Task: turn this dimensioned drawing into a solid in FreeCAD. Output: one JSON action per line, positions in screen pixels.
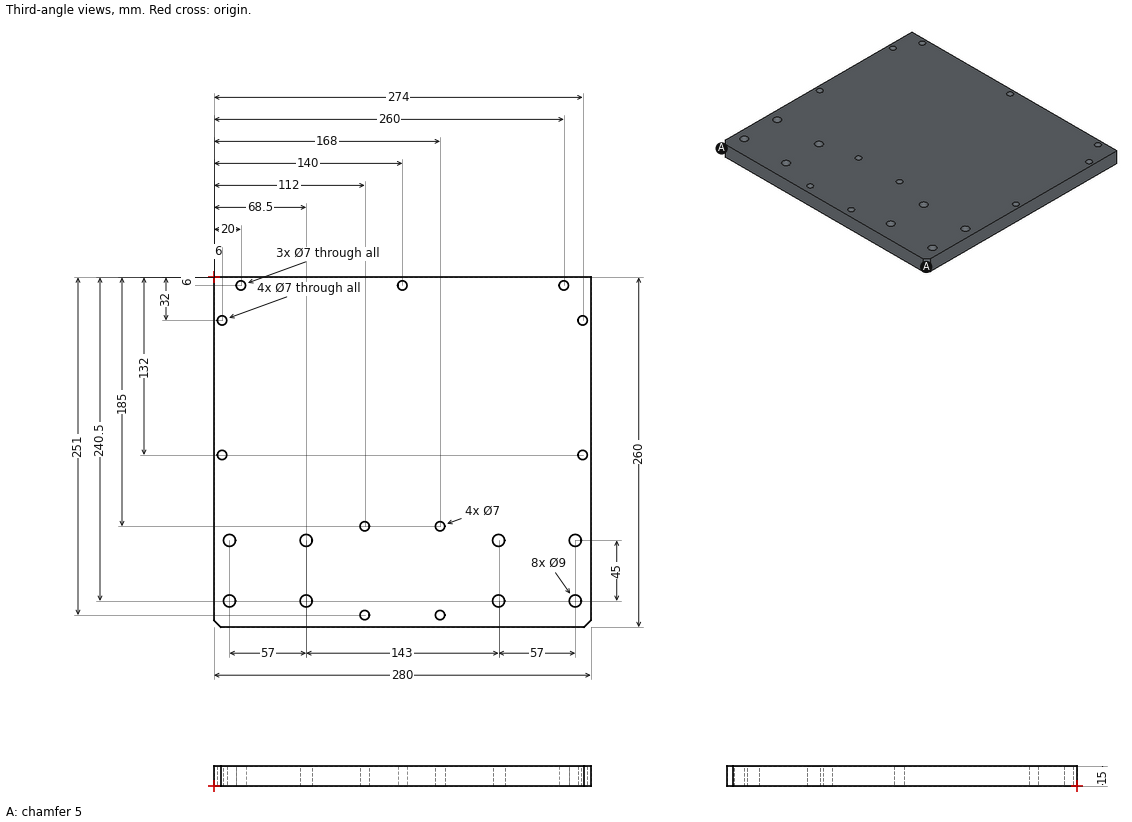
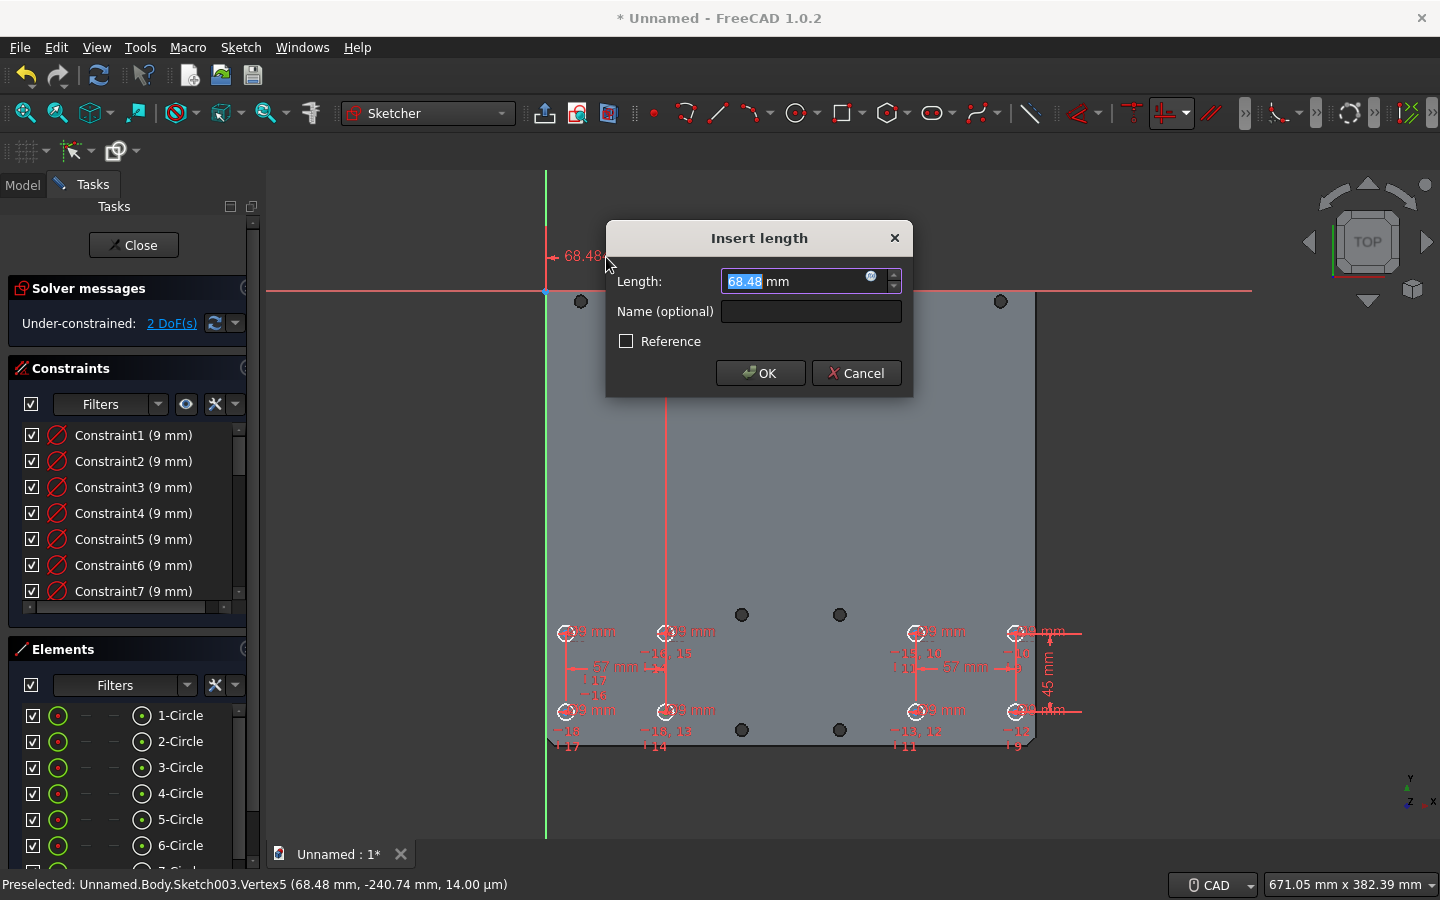
{"action": "type", "text": "68.5"}
{"action": "key", "text": "Return"}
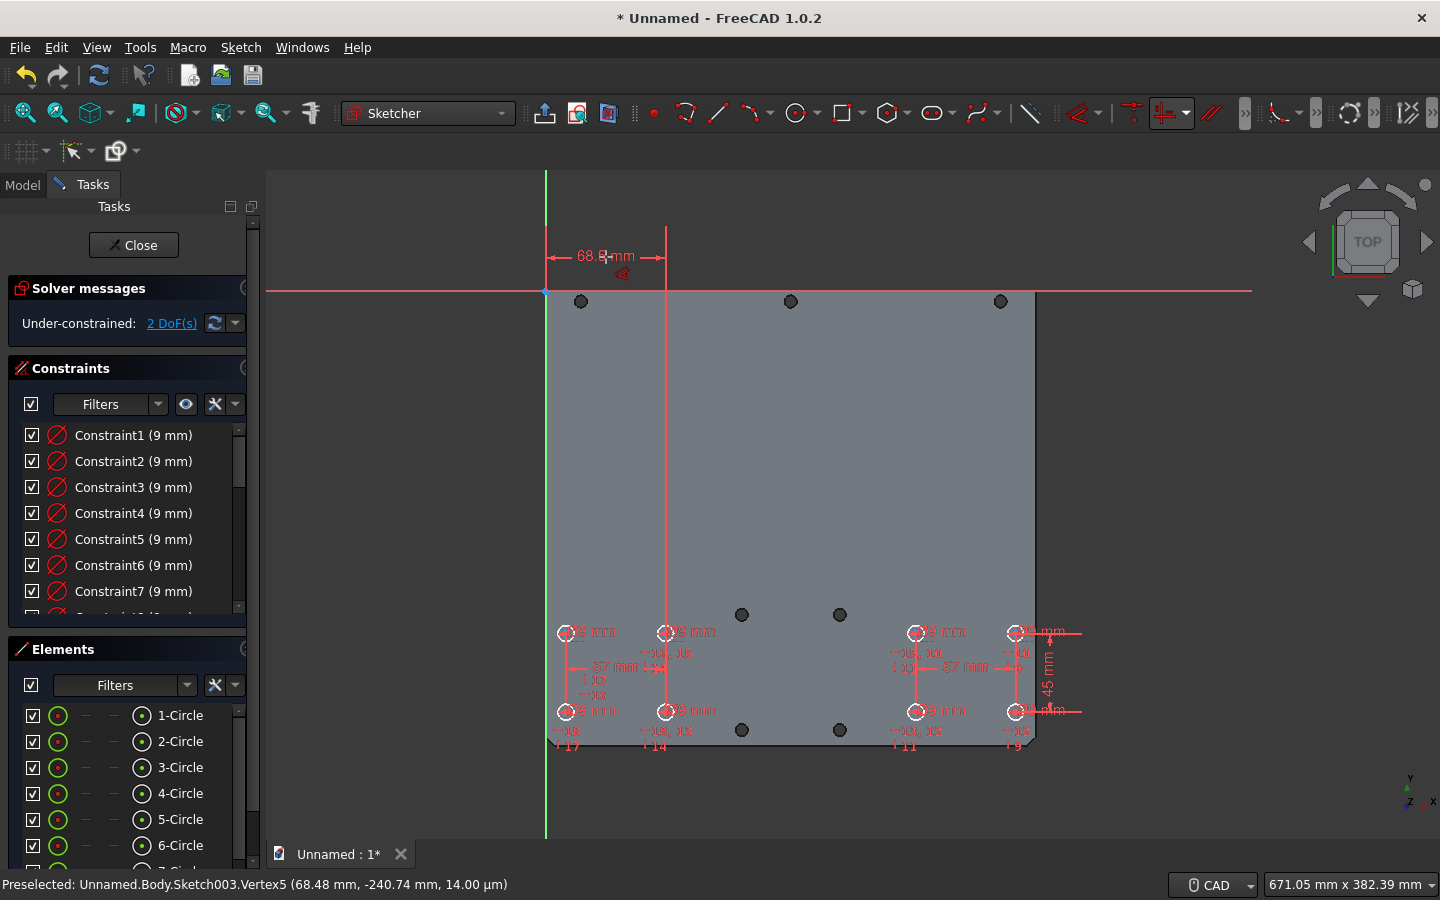
{"action": "left_click", "coordinate": [916, 712]}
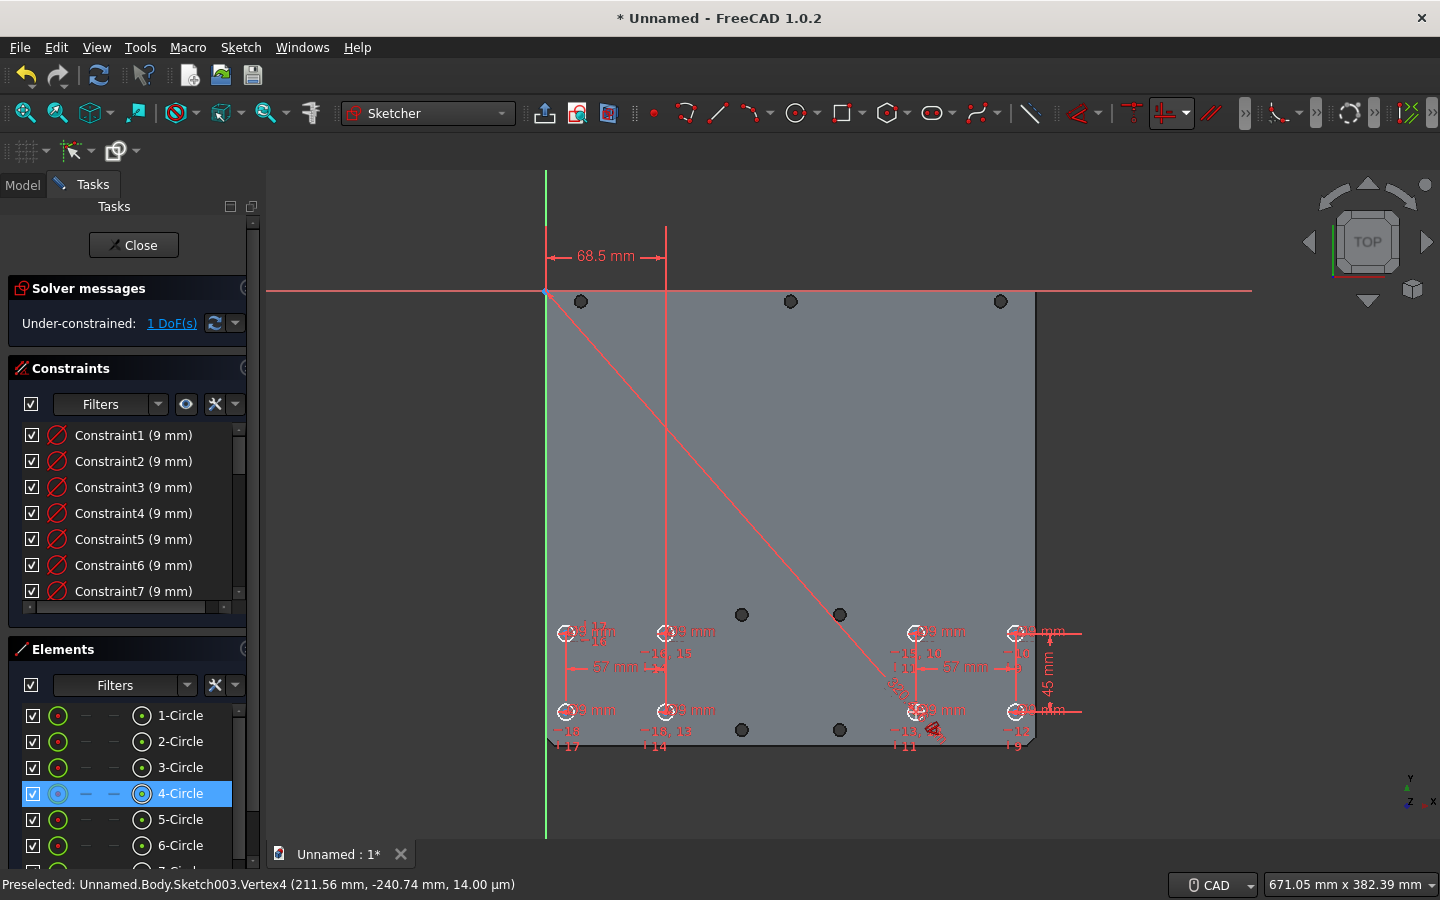
{"action": "left_click", "coordinate": [666, 712]}
{"action": "left_click", "coordinate": [791, 746]}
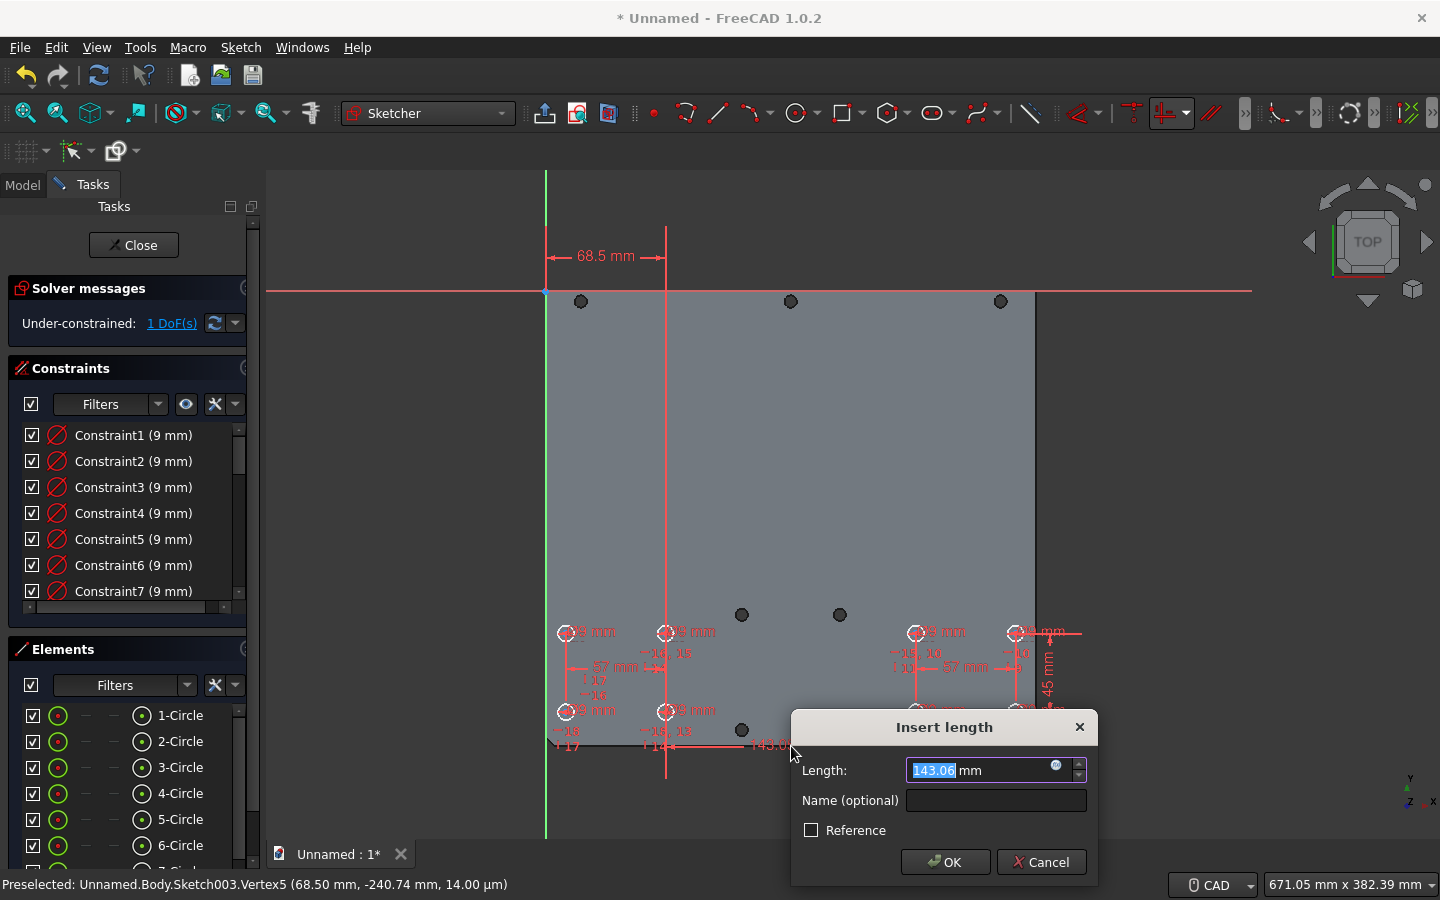
{"action": "type", "text": "143"}
{"action": "key", "text": "Return"}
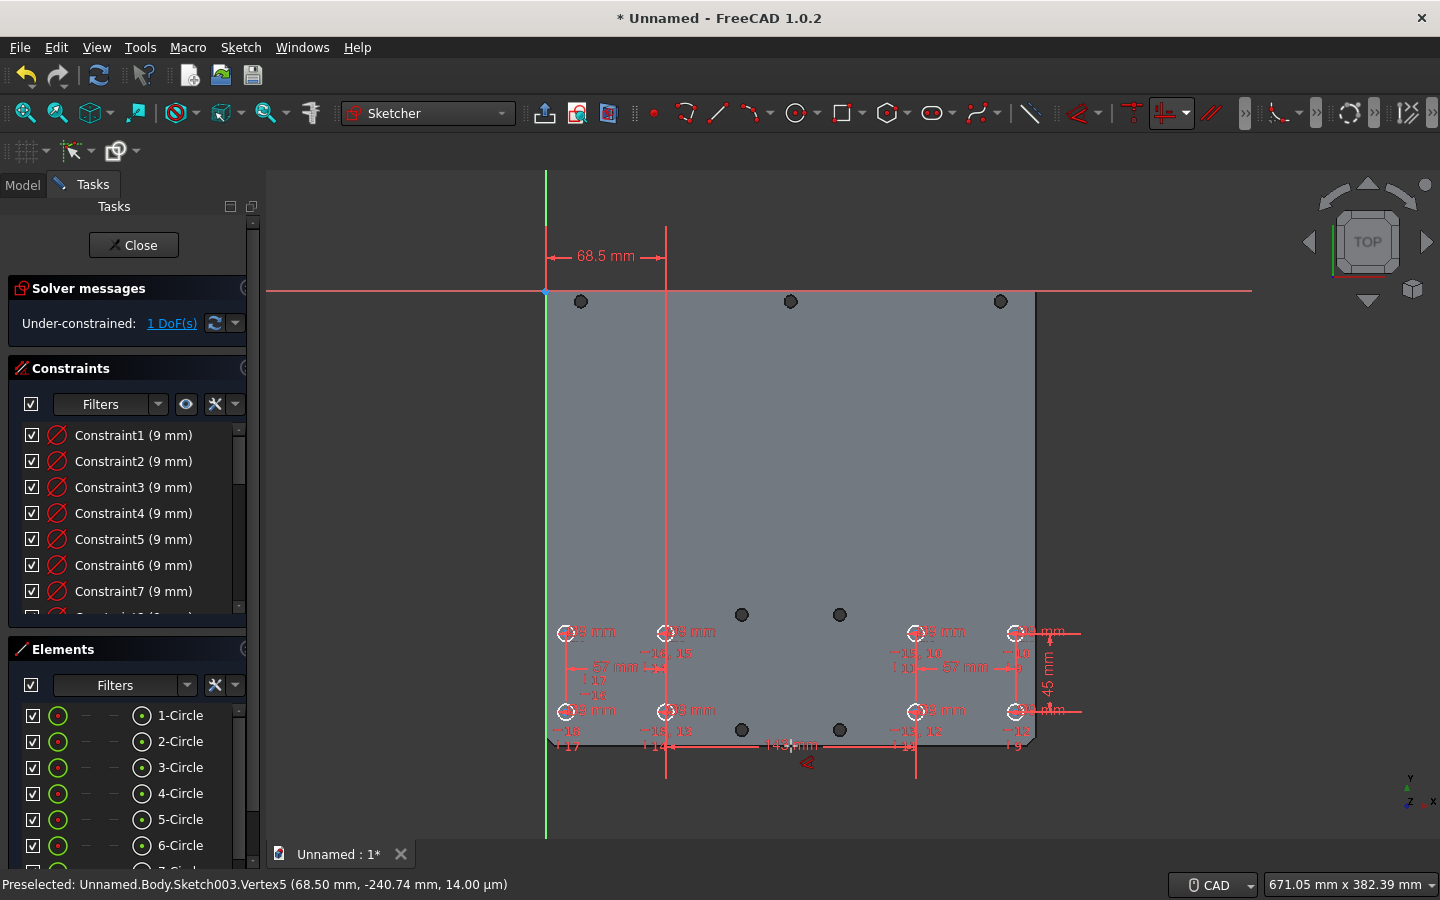
{"action": "left_click", "coordinate": [1016, 712]}
{"action": "left_click", "coordinate": [512, 502]}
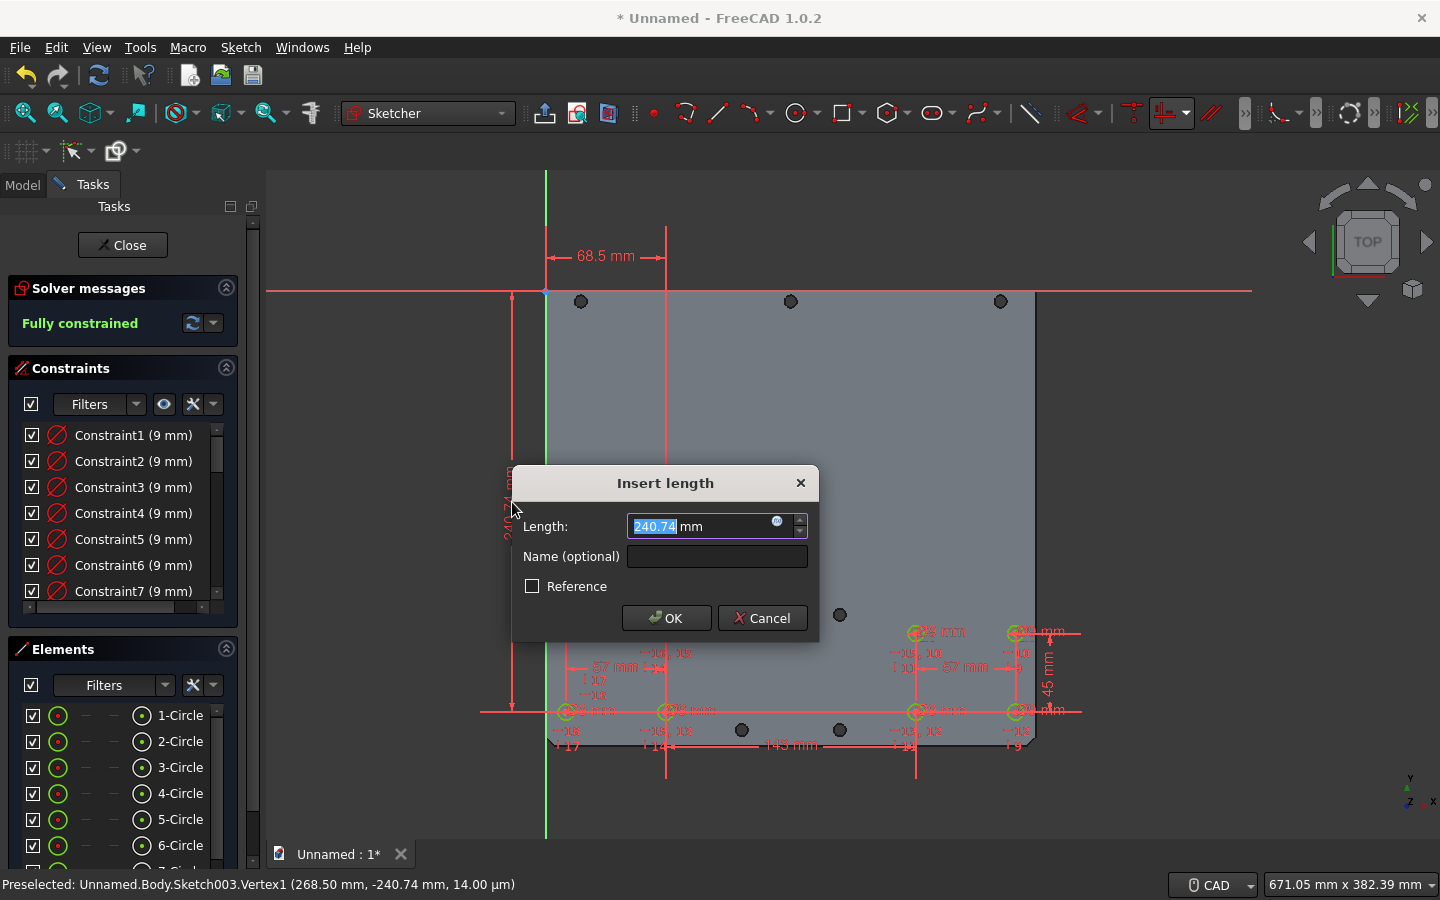
{"action": "type", "text": "240.5"}
{"action": "key", "text": "Return"}
{"action": "key", "text": "Escape"}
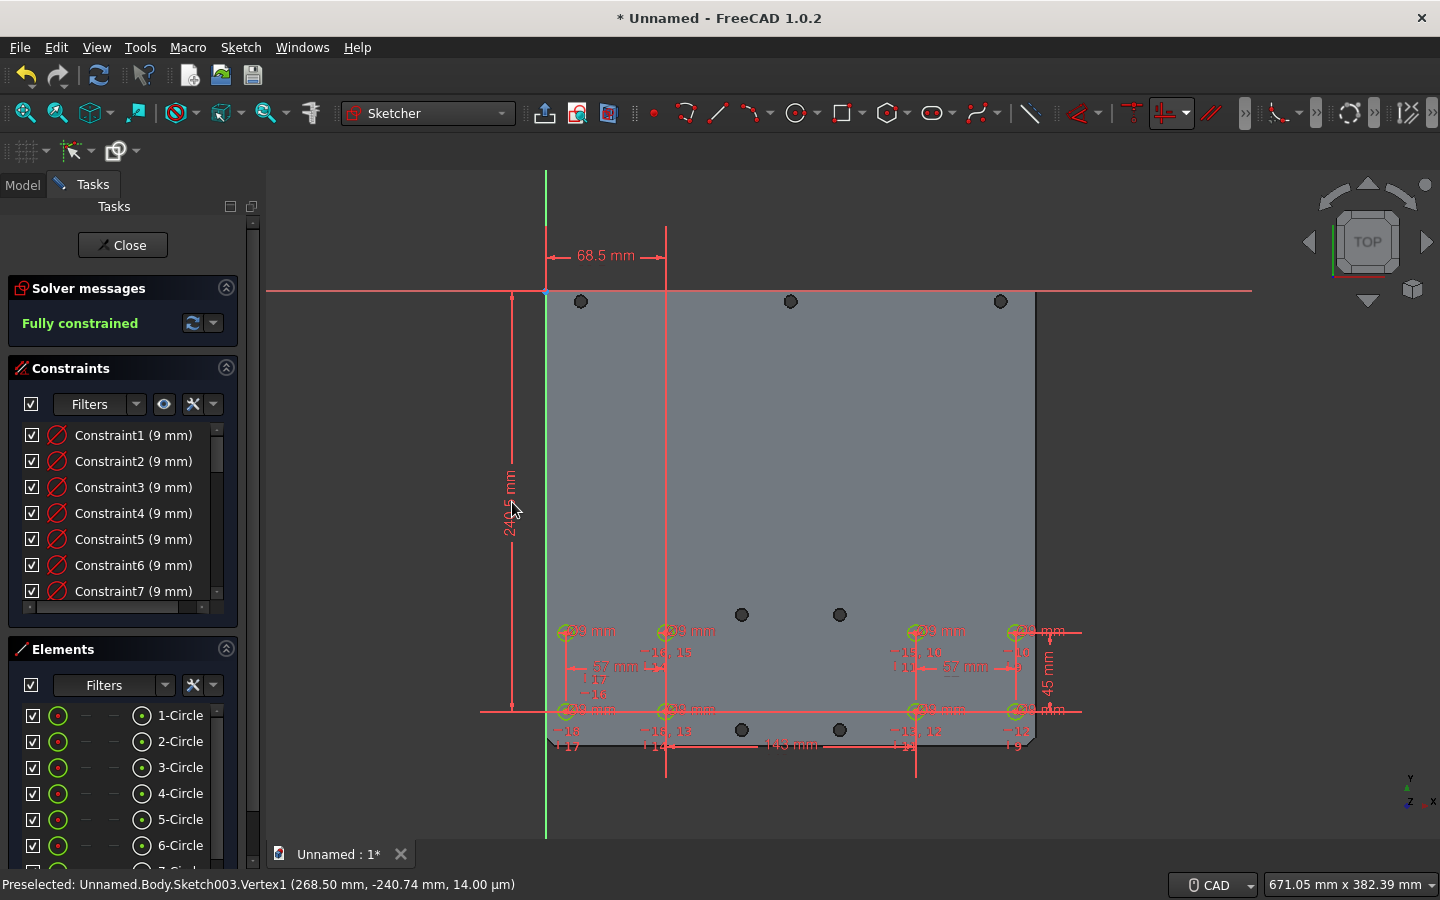
{"action": "left_click", "coordinate": [123, 245]}